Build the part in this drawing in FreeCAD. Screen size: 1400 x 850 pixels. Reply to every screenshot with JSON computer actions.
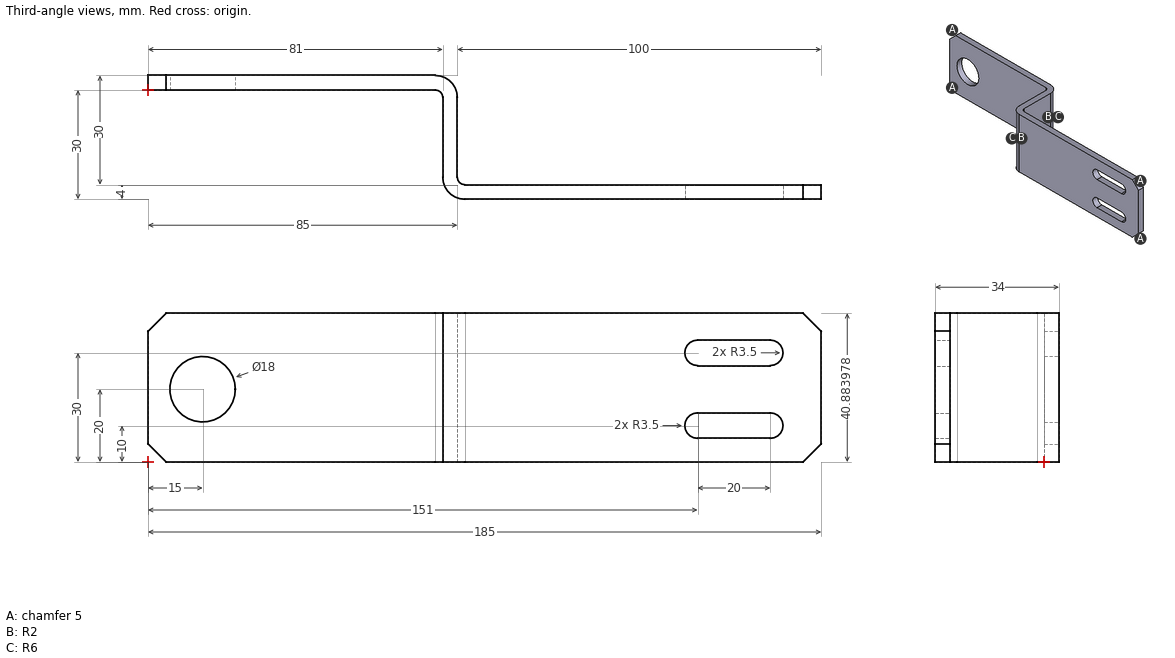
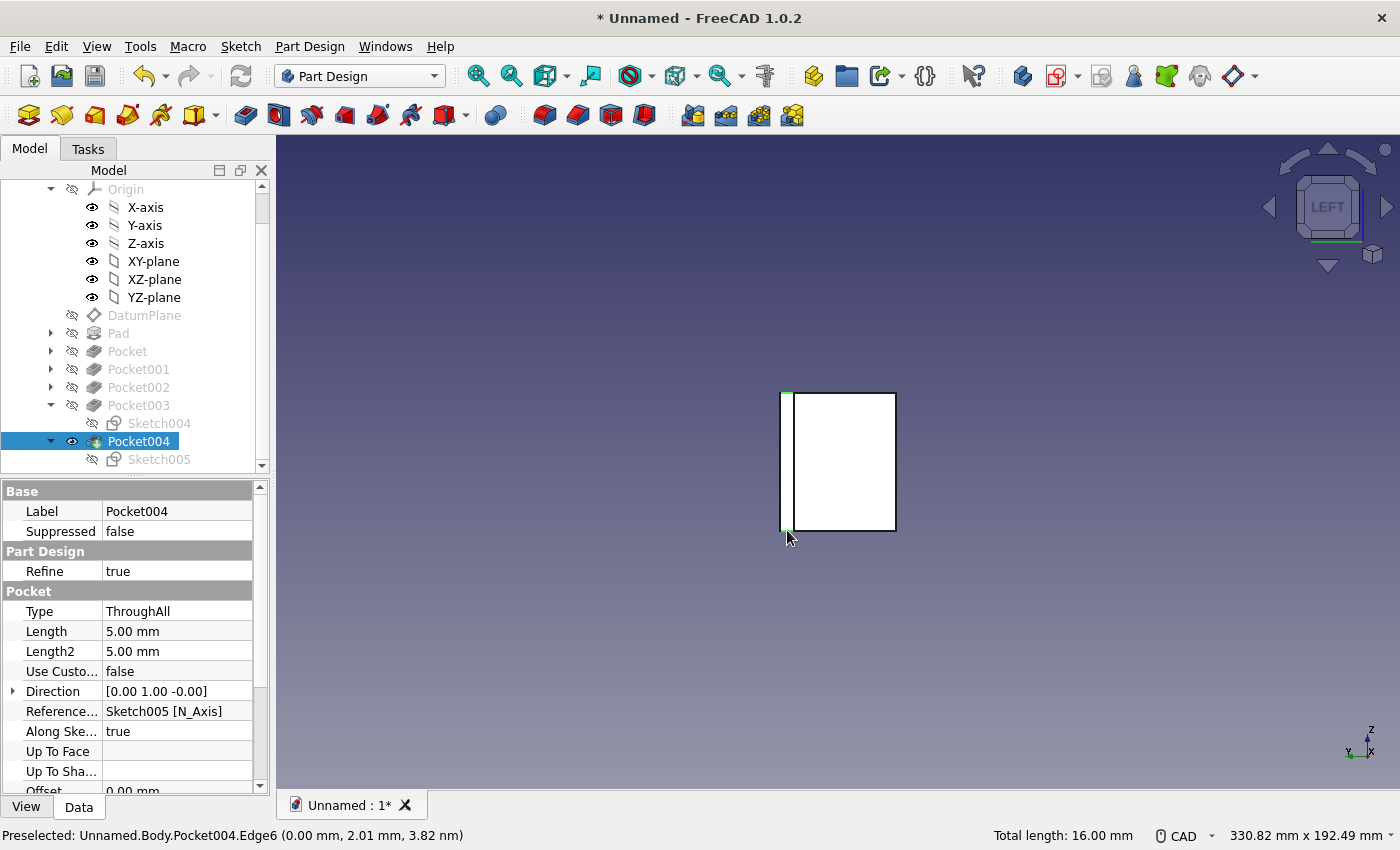
{"action": "left_click", "coordinate": [578, 116]}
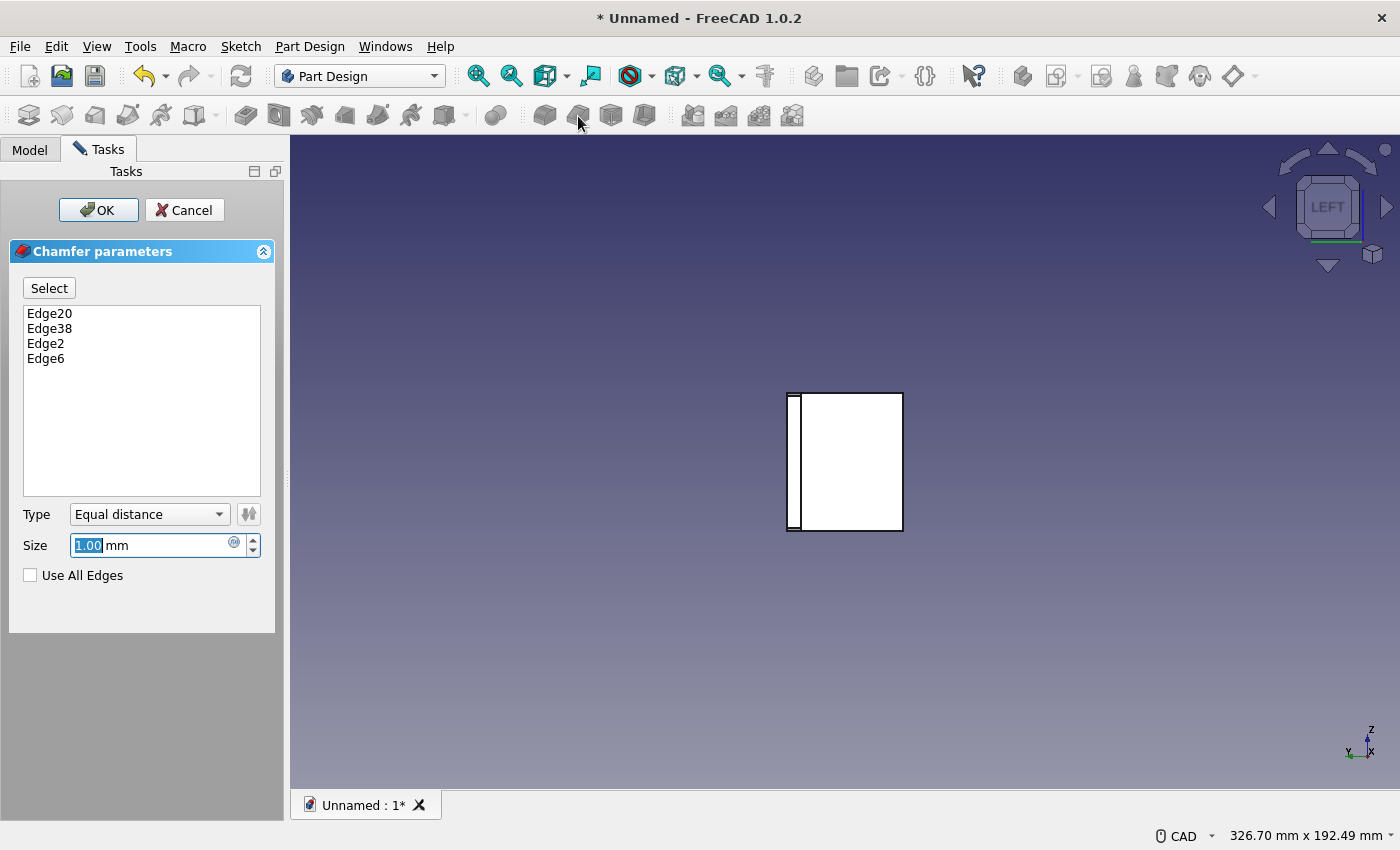
{"action": "type", "text": "5"}
{"action": "key", "text": "Tab"}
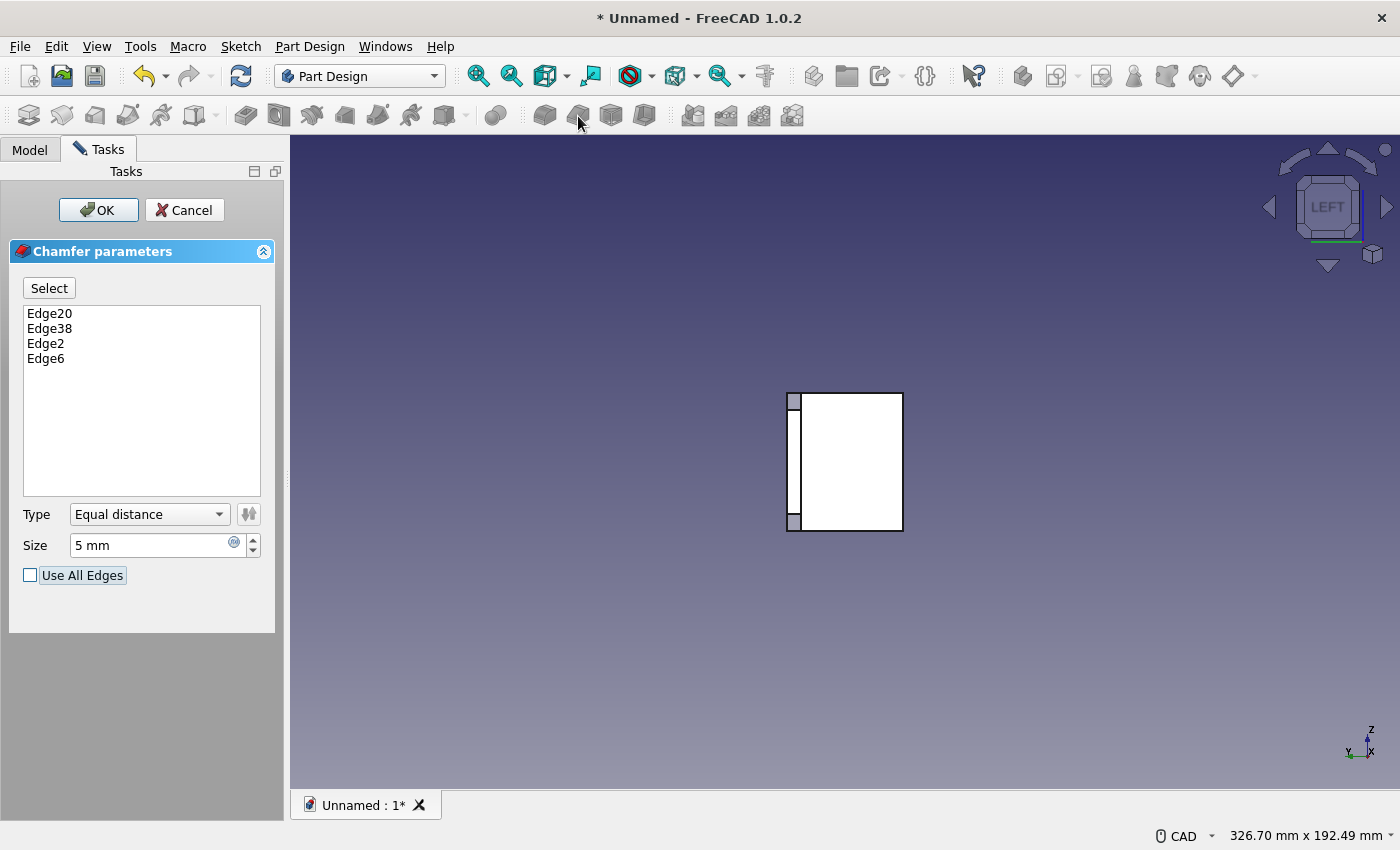
{"action": "left_click", "coordinate": [99, 210]}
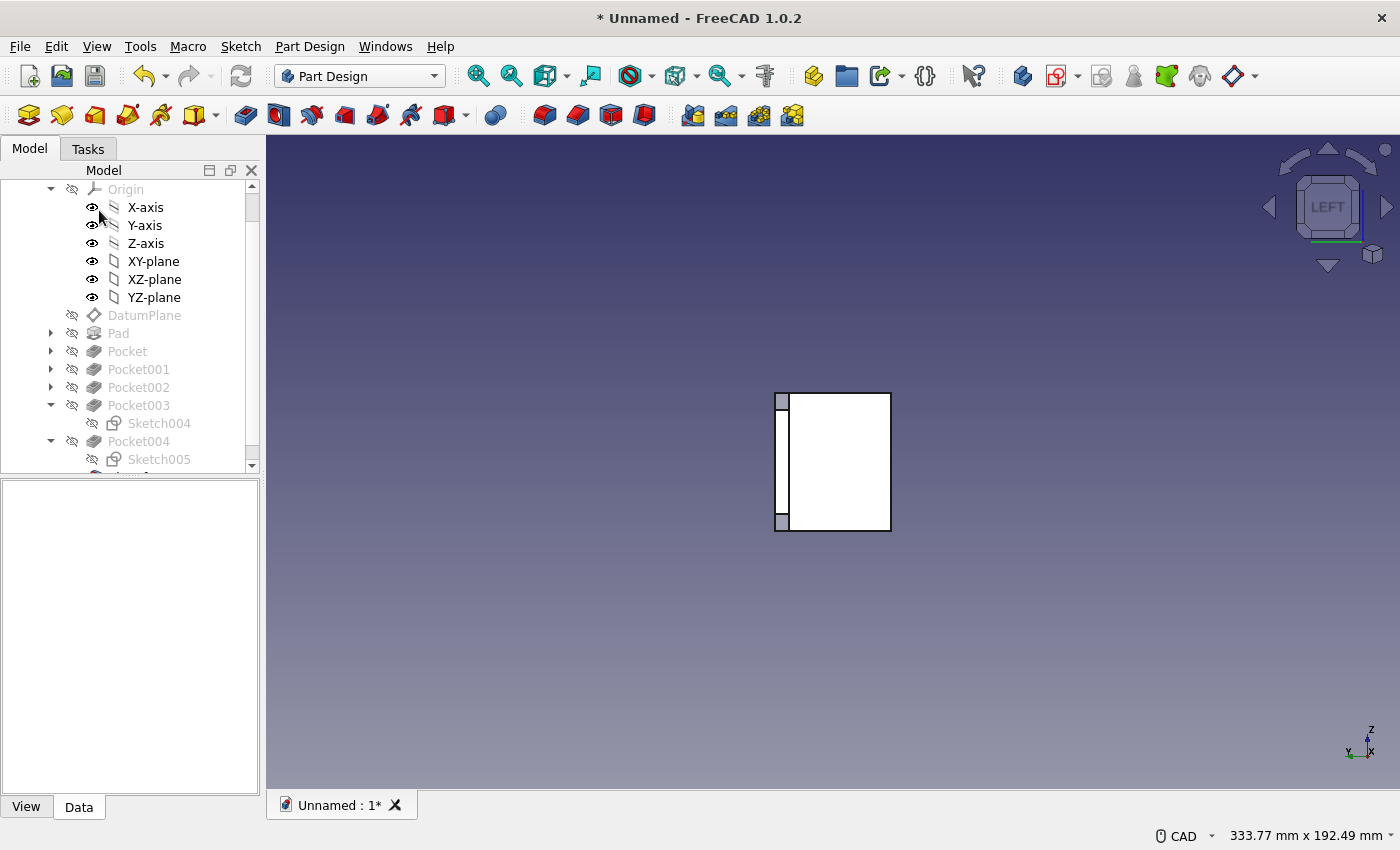
{"action": "key", "text": "v f"}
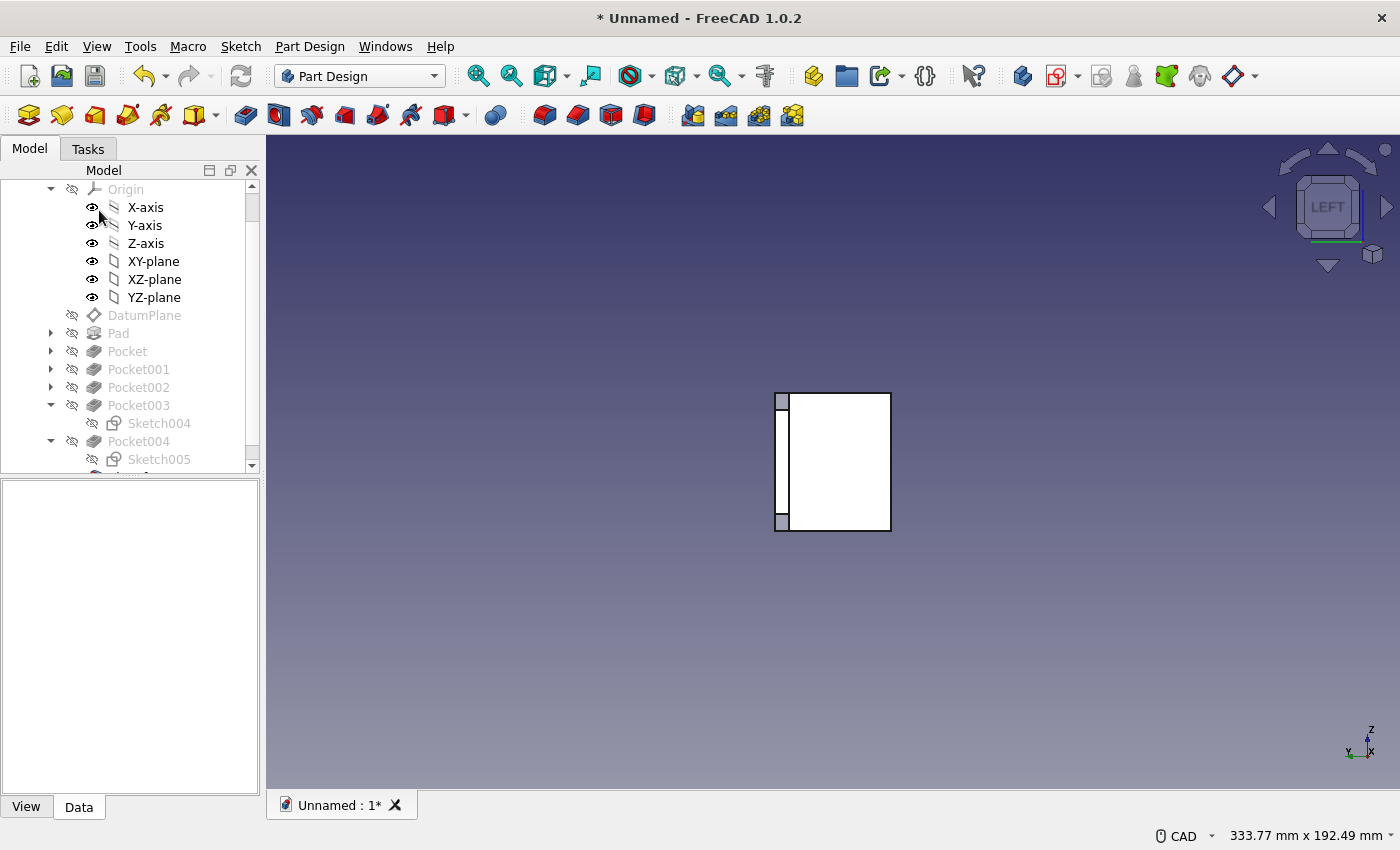
{"action": "key", "text": "0"}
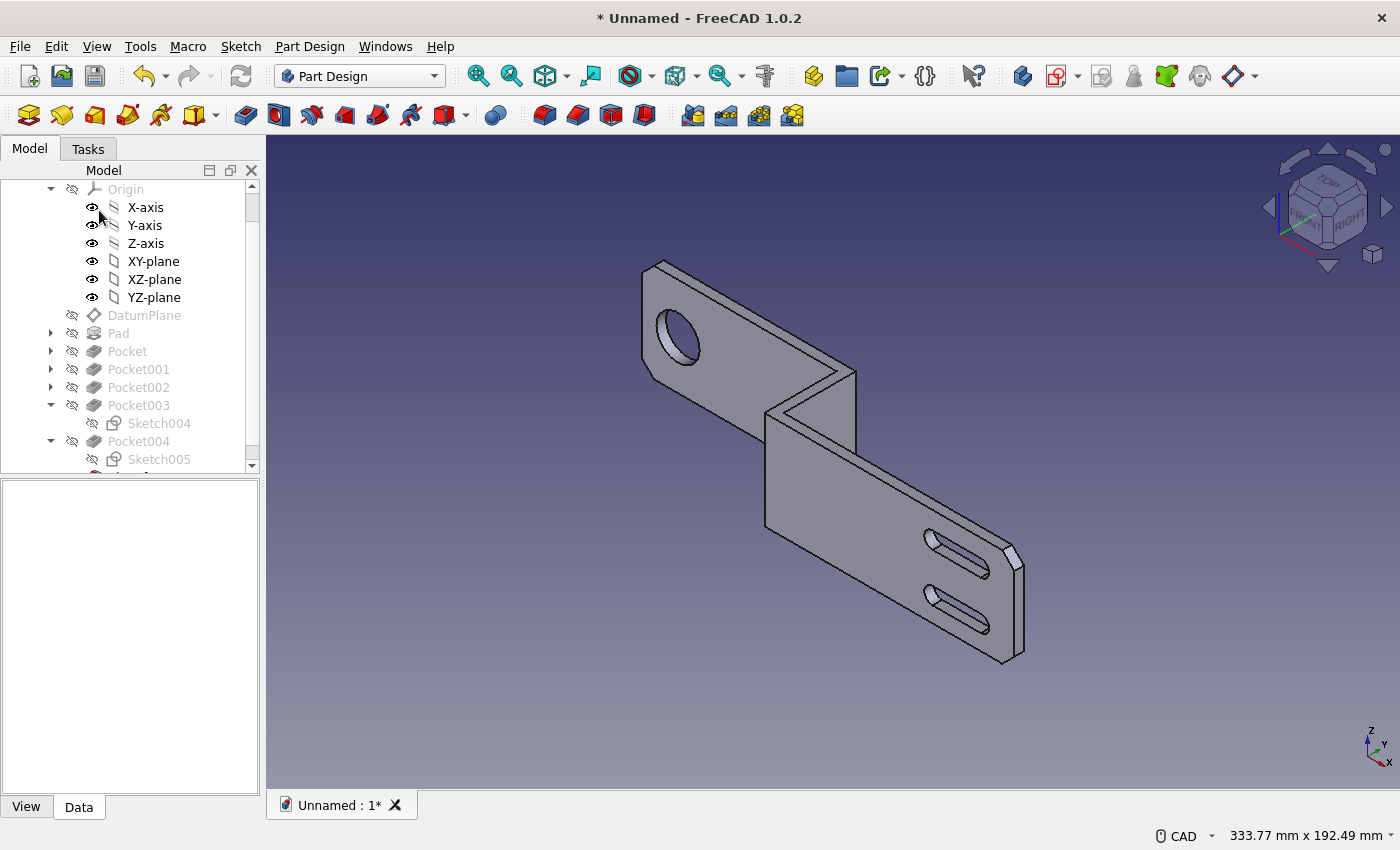
{"action": "key", "text": "2"}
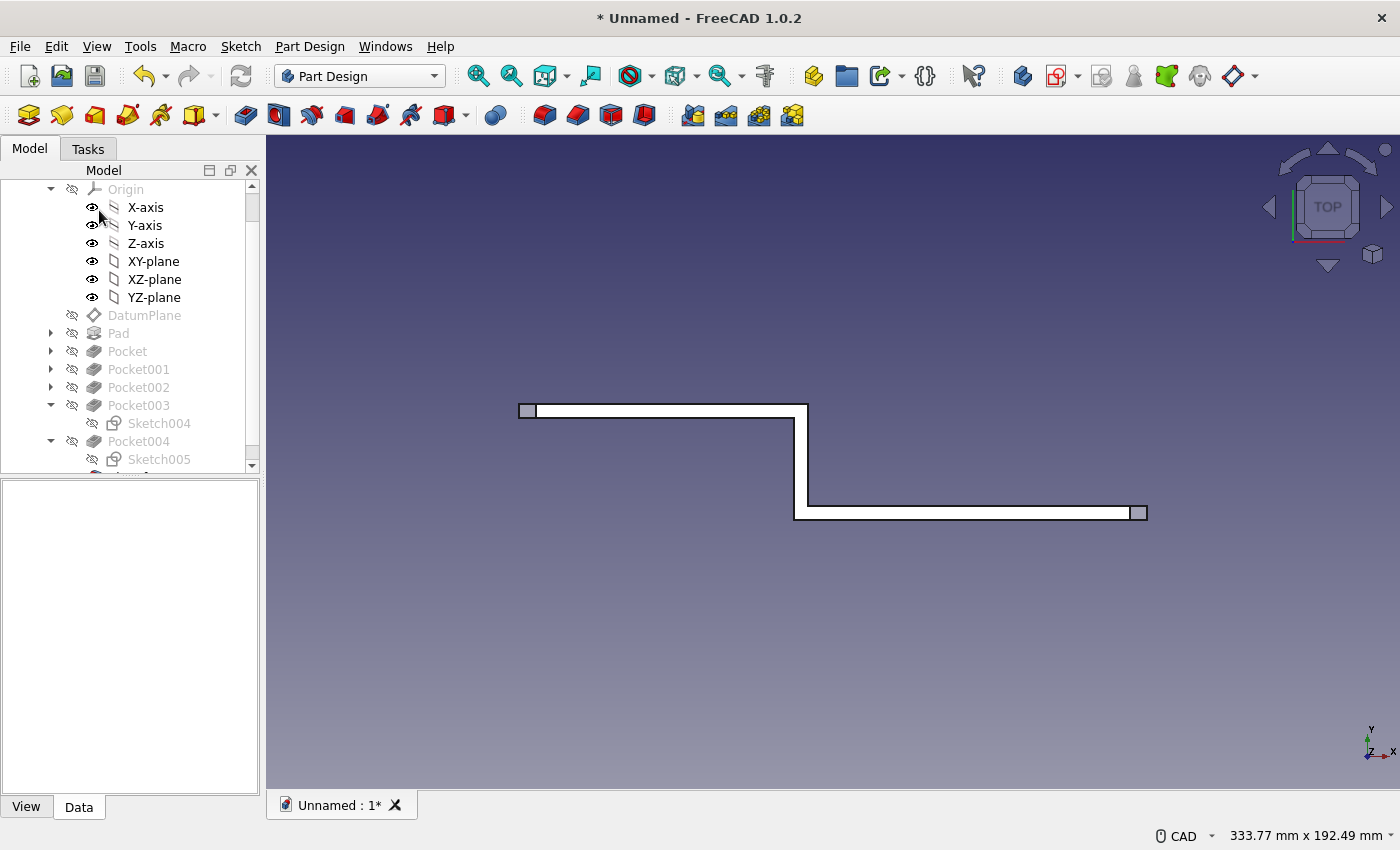
{"action": "key", "text": "1"}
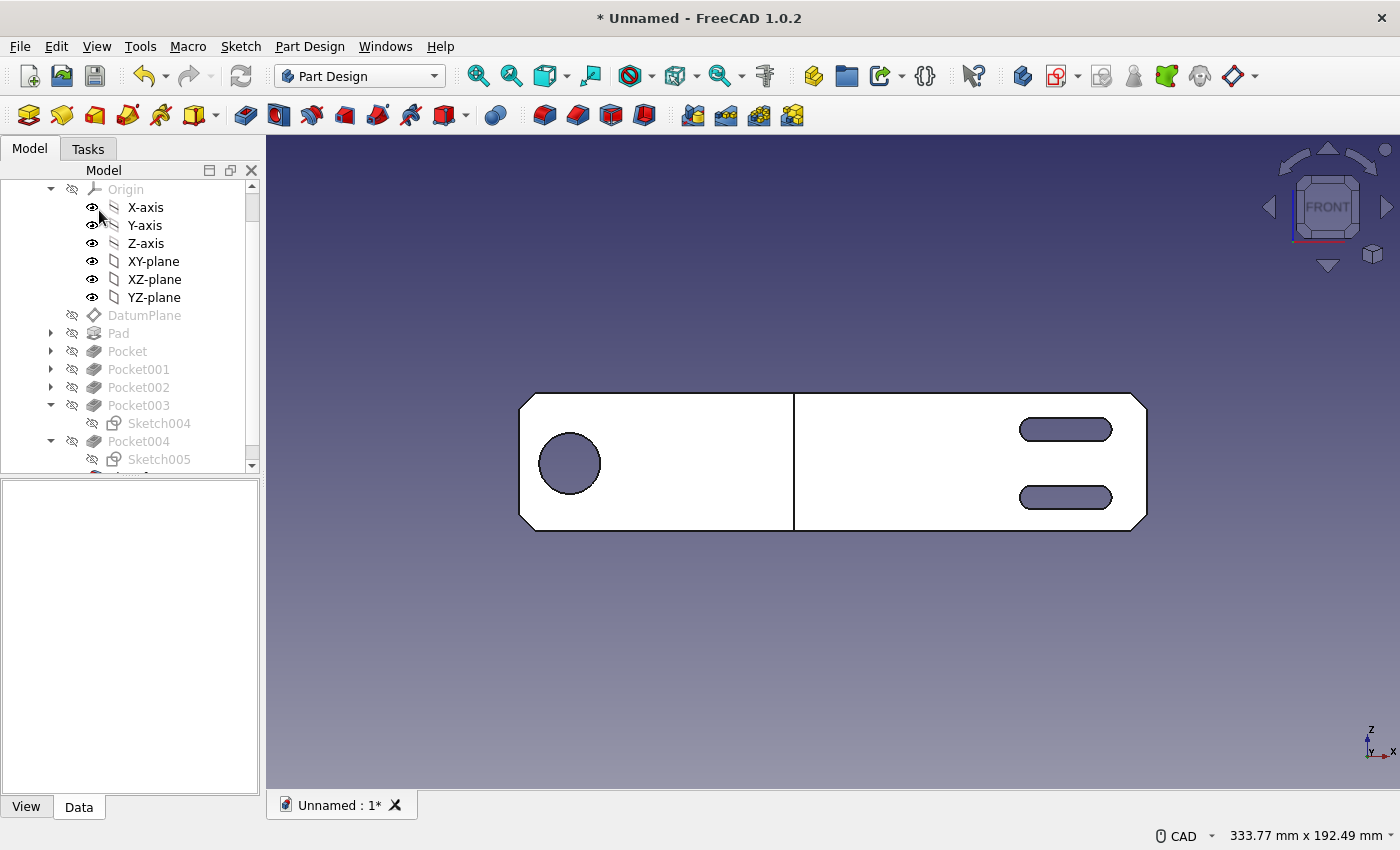
{"action": "key", "text": "3"}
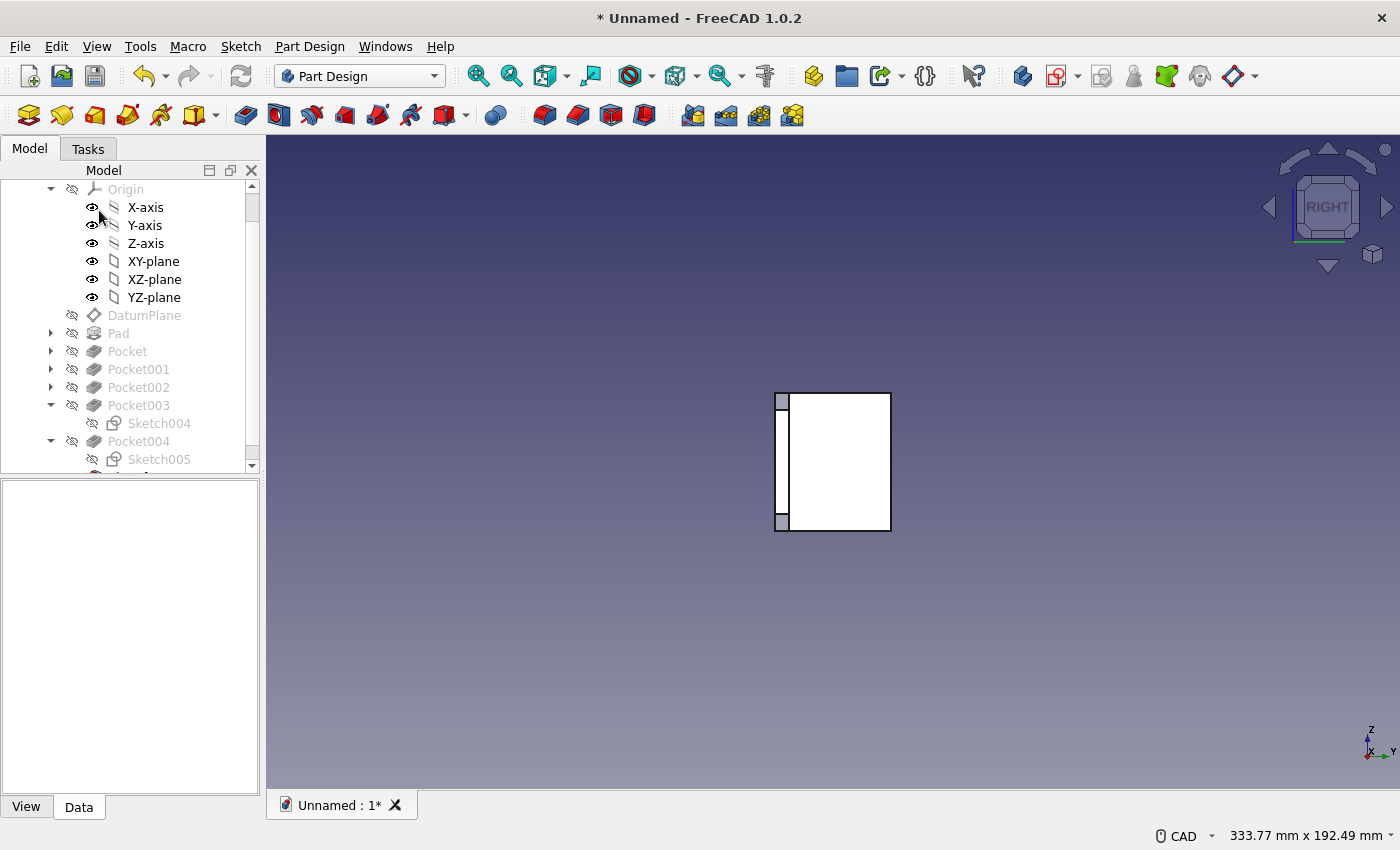
{"action": "left_click", "coordinate": [479, 76]}